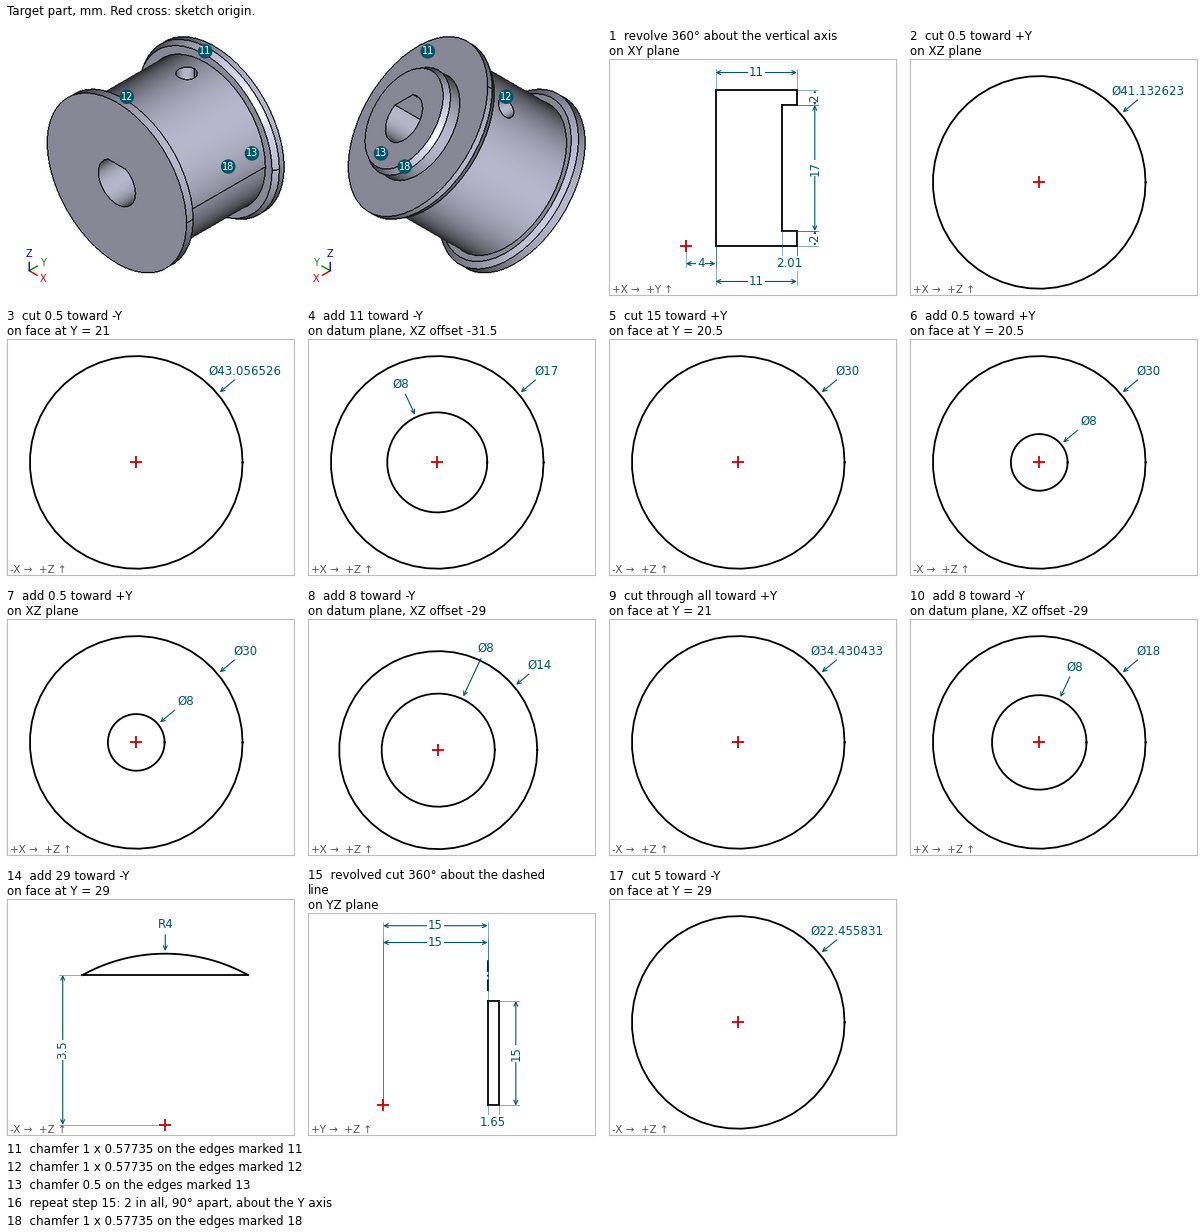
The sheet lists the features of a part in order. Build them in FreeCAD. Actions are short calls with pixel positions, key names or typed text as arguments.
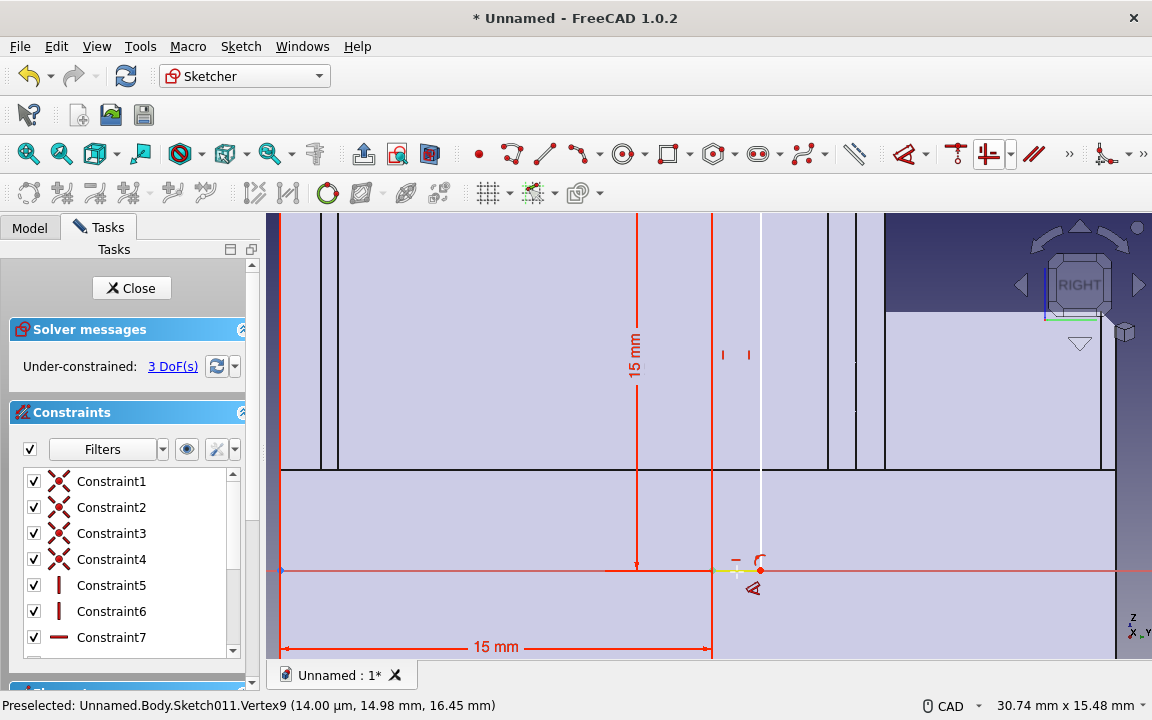
click(737, 571)
click(737, 605)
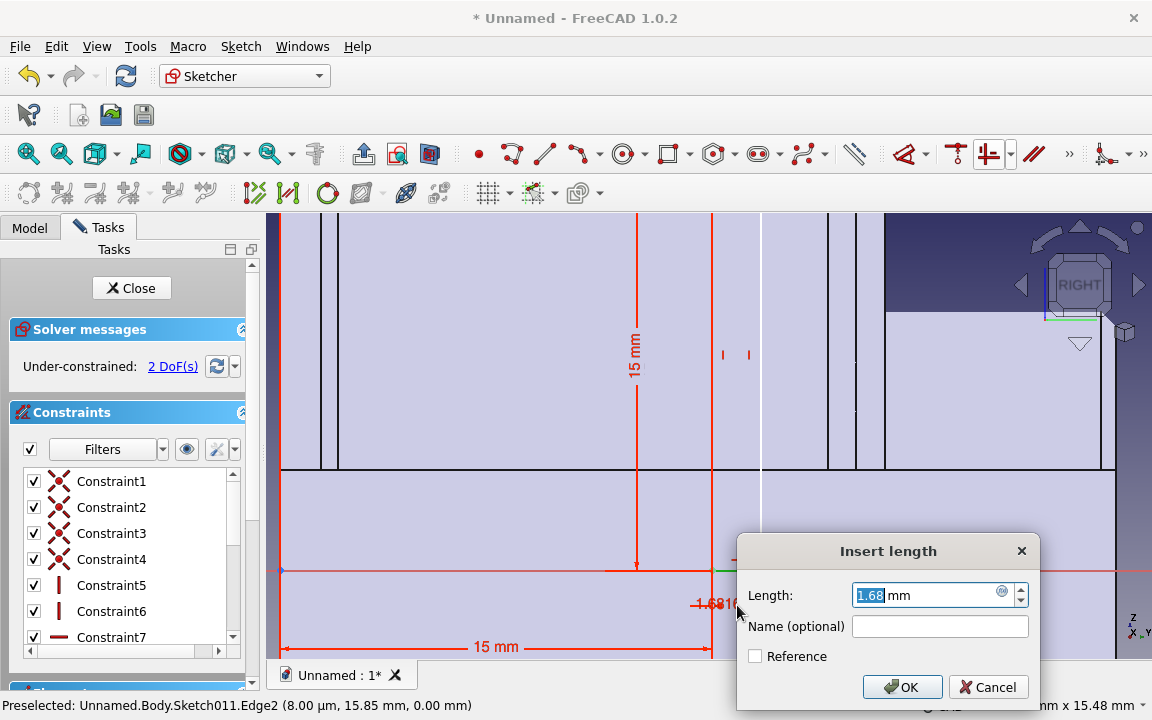
text(1.65)
key(Return)
key(Escape)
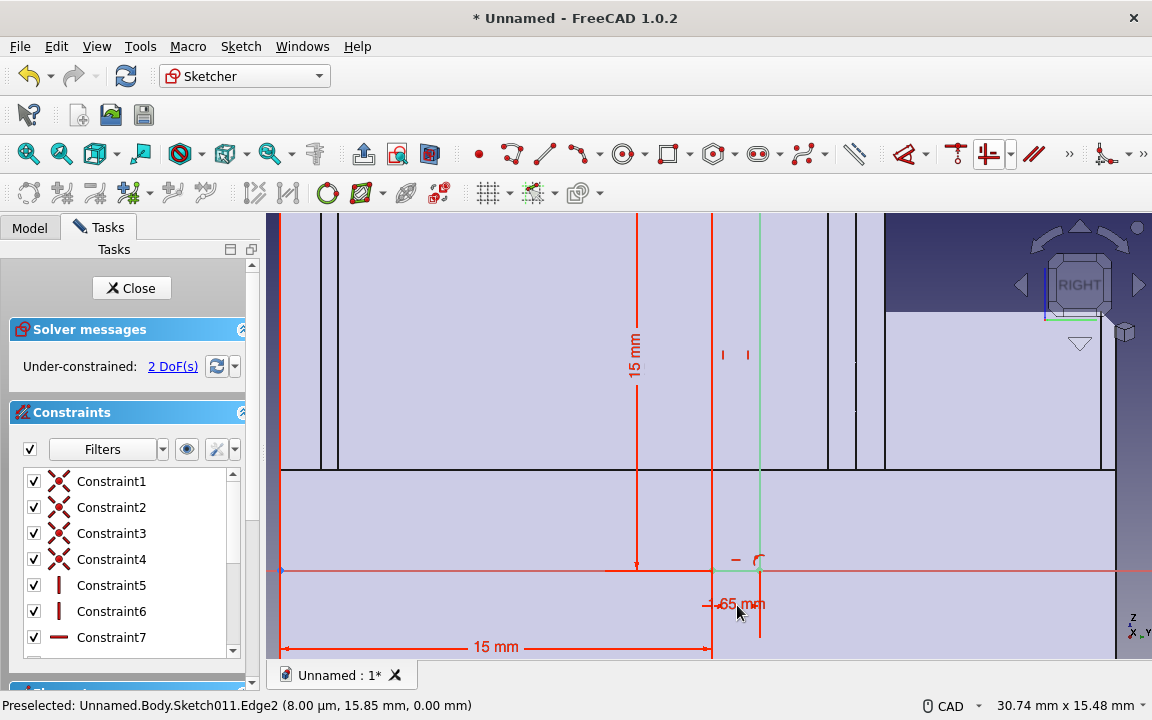
click(132, 288)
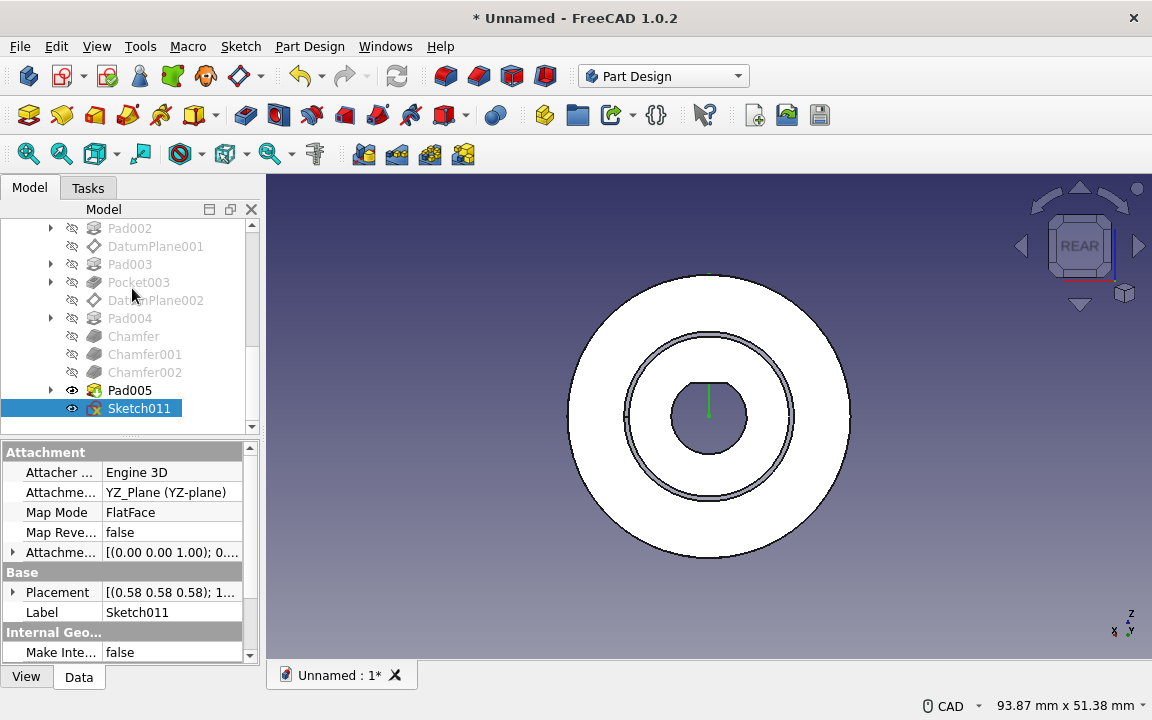
click(312, 116)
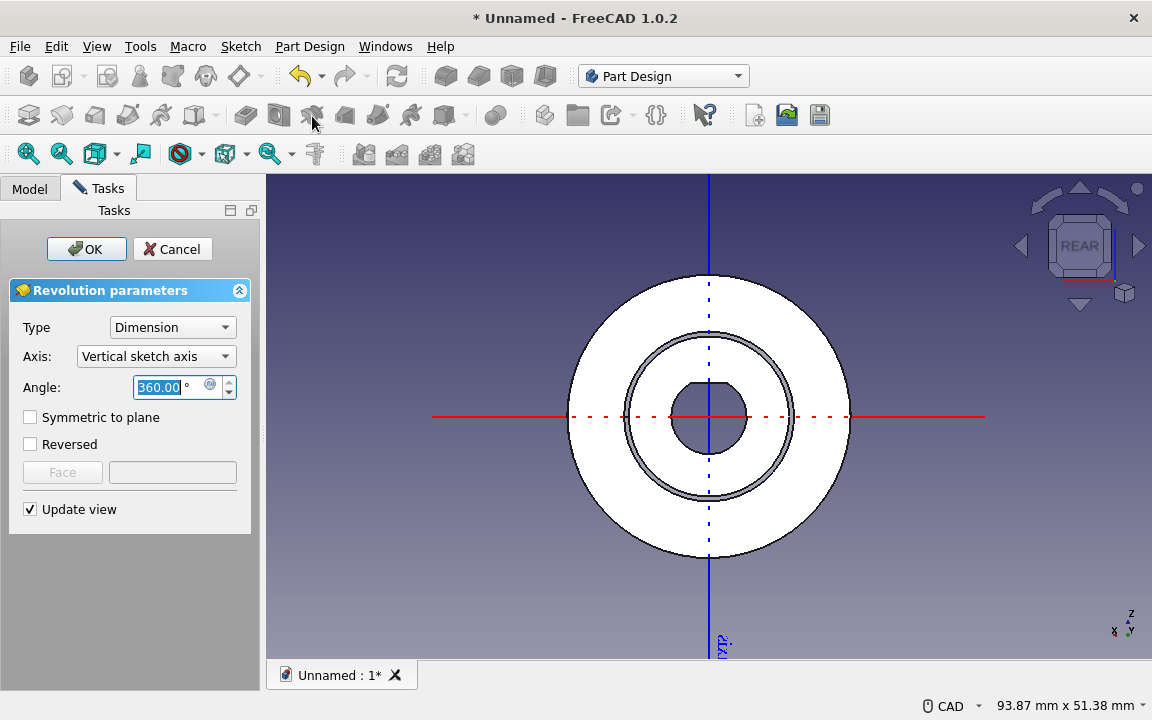
click(157, 356)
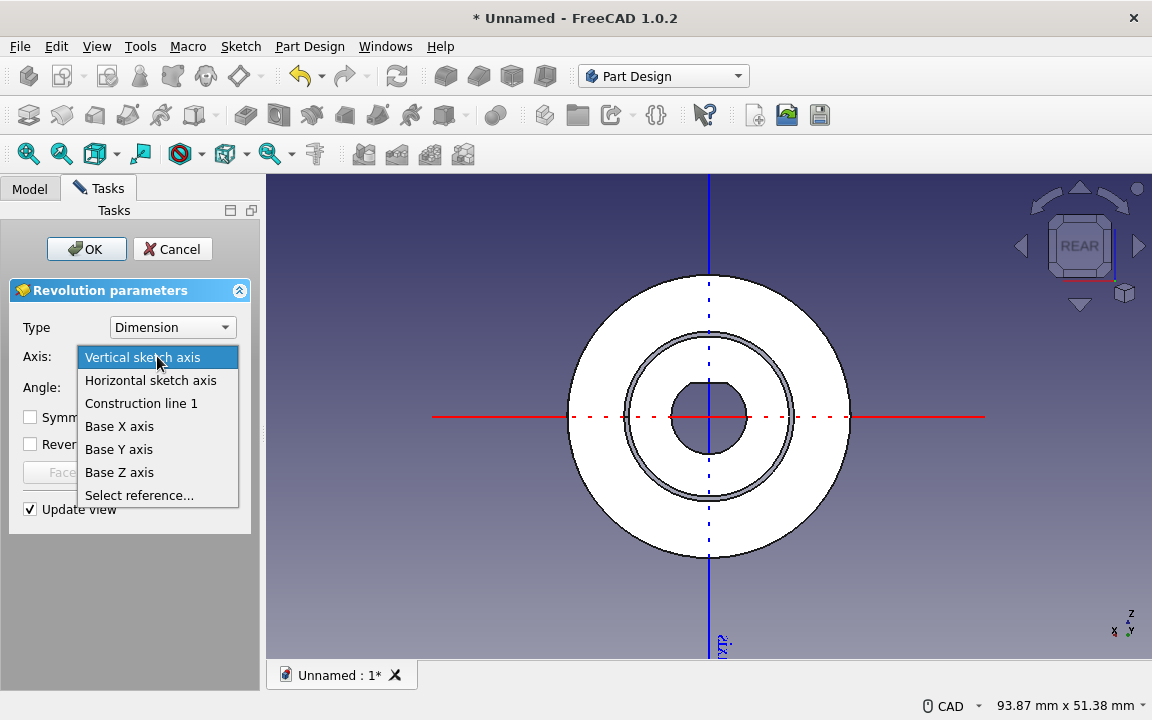
click(156, 404)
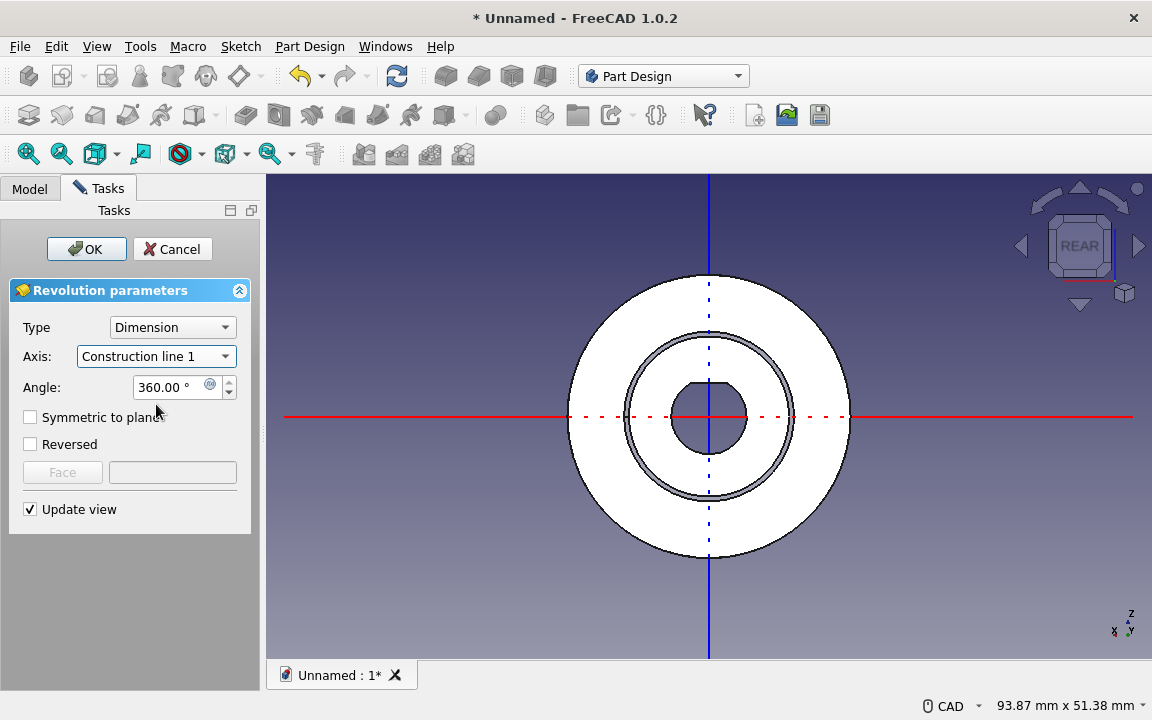
click(87, 249)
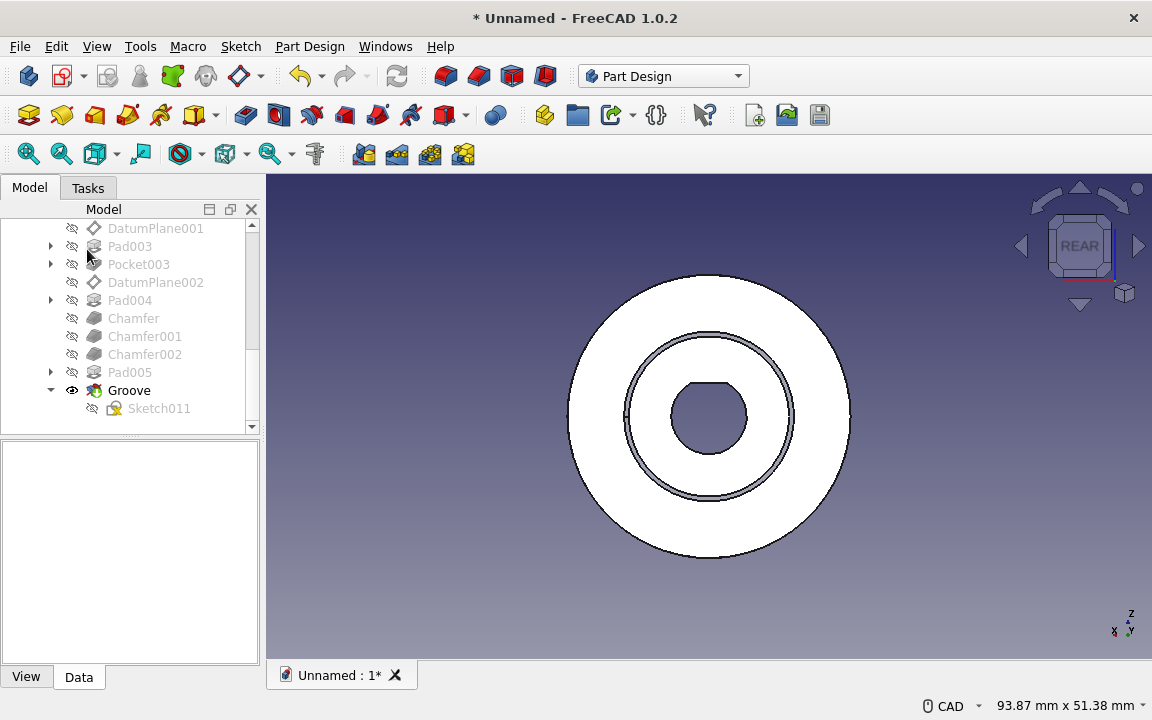
click(117, 390)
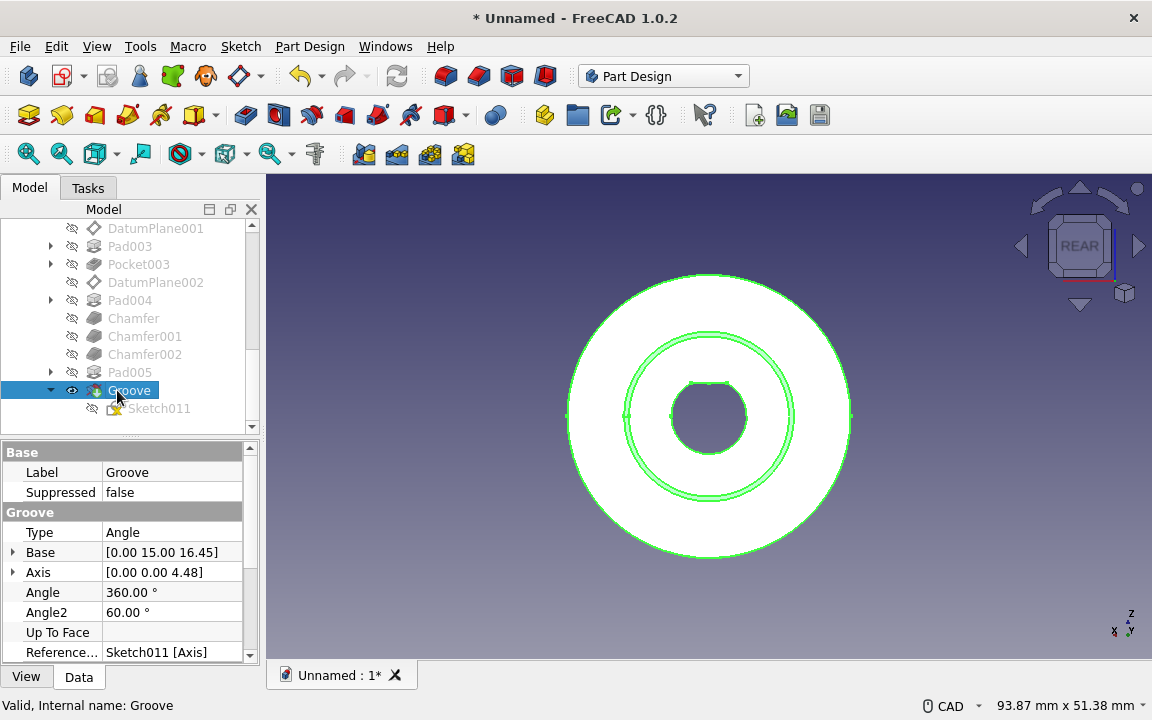
click(430, 154)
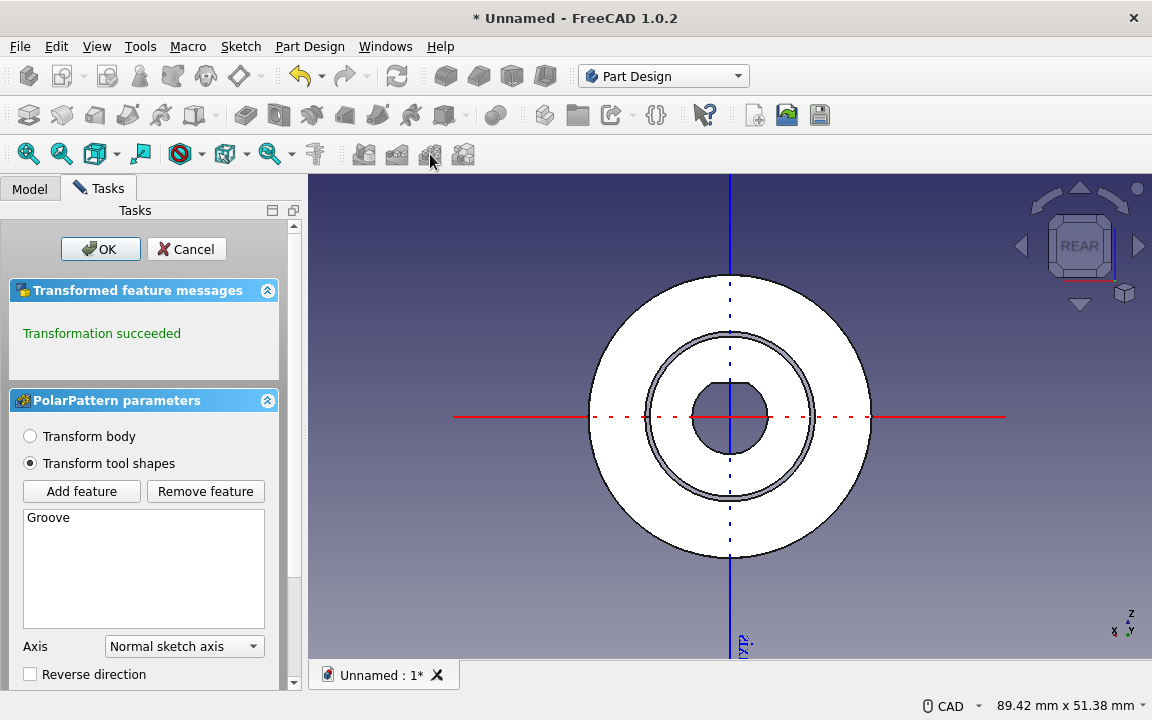
click(185, 646)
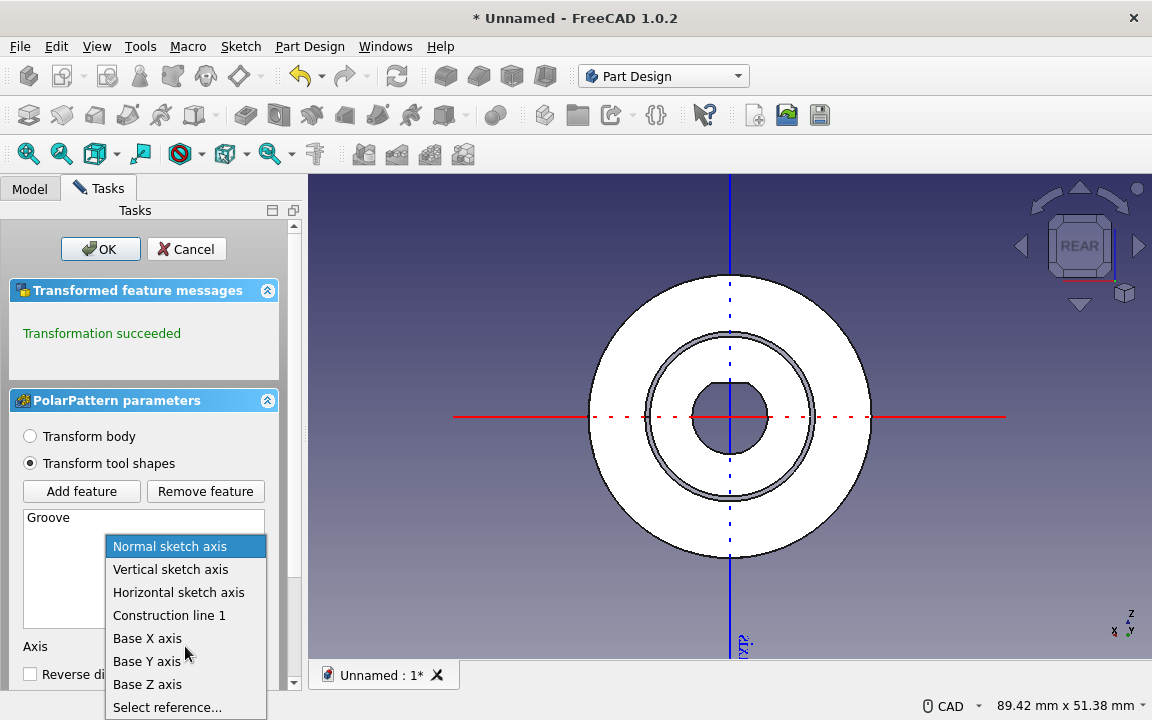
click(184, 662)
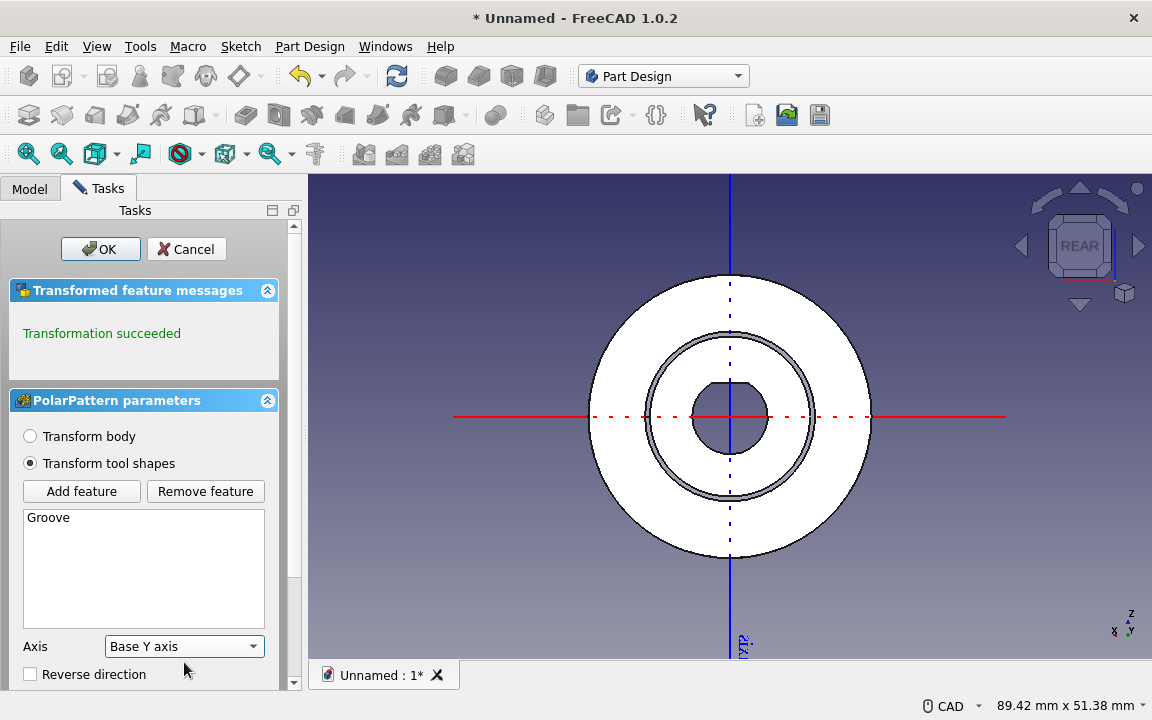
scroll(294, 455, down, 2)